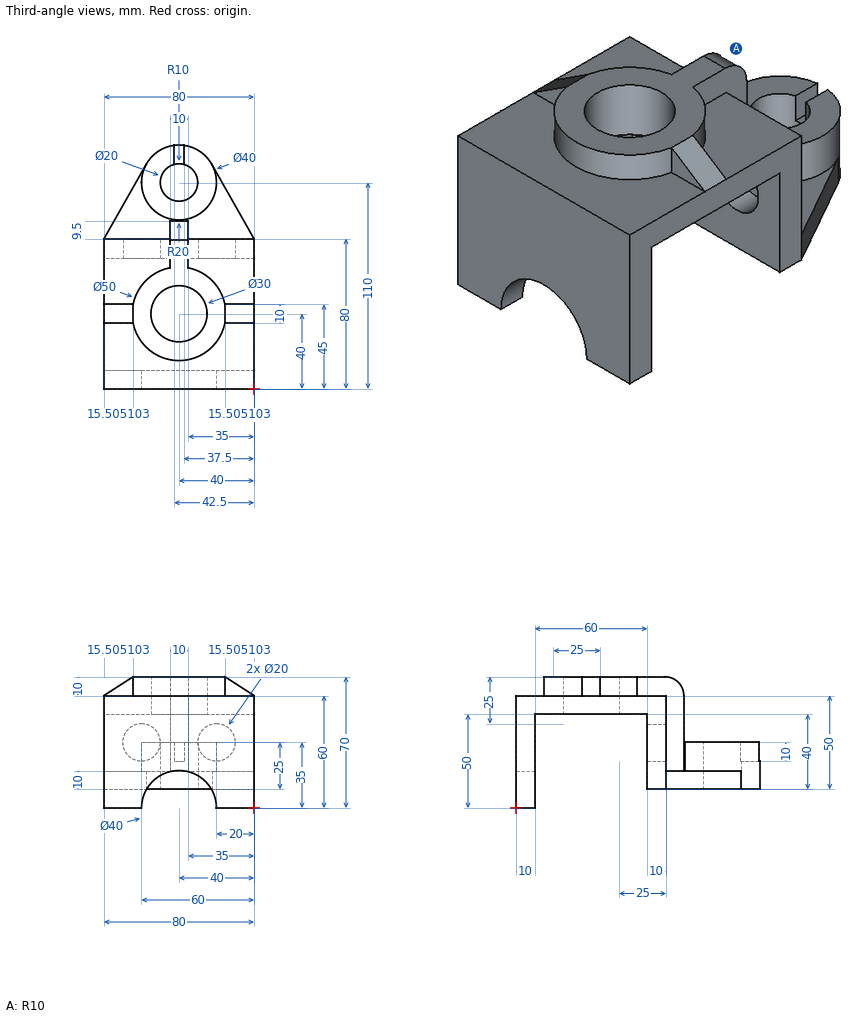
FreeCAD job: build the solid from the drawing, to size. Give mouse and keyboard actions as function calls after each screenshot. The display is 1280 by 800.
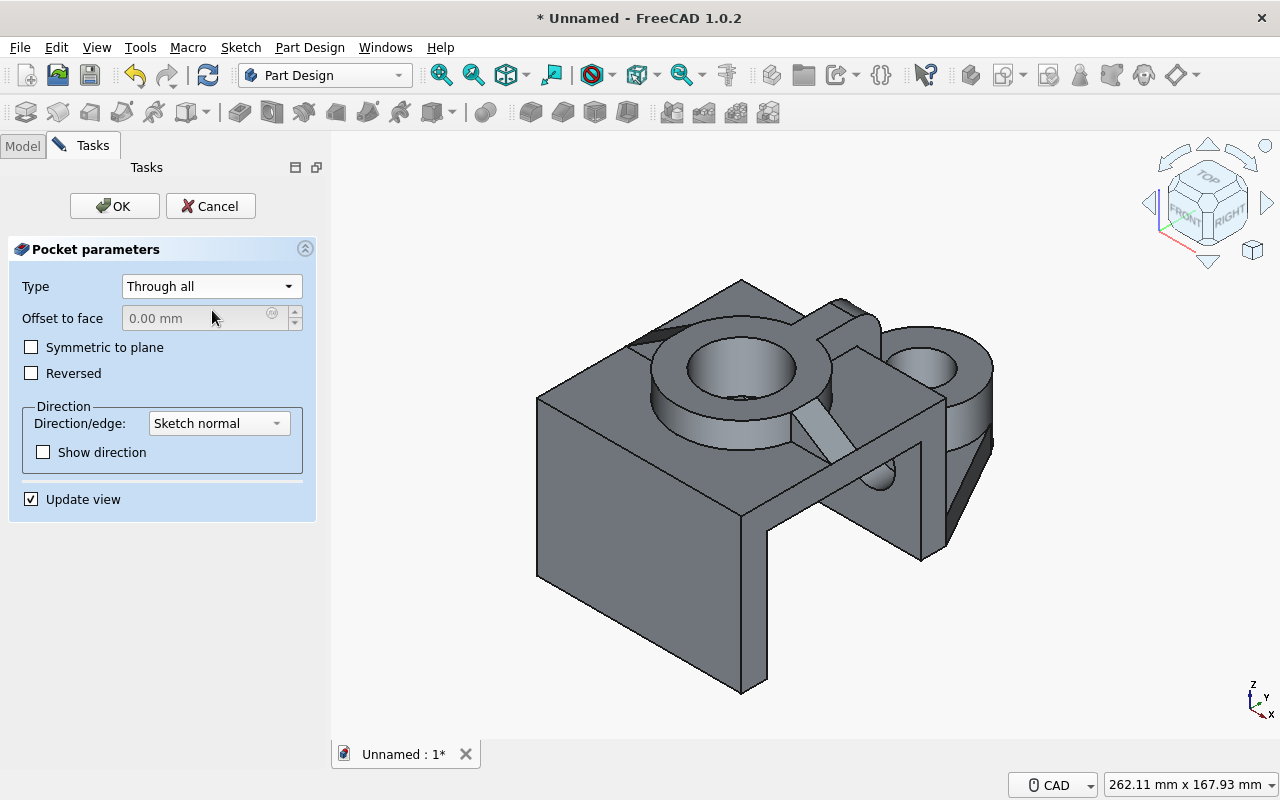
click(115, 206)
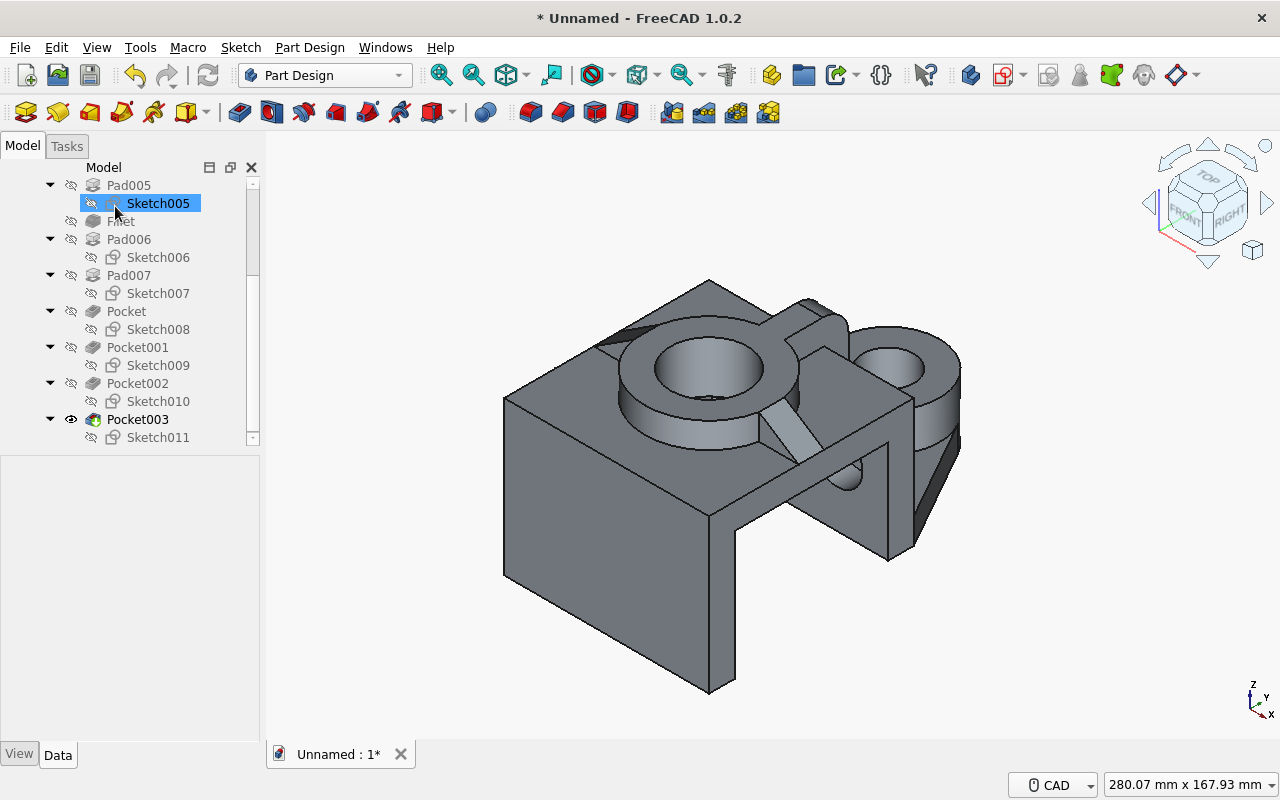
click(888, 334)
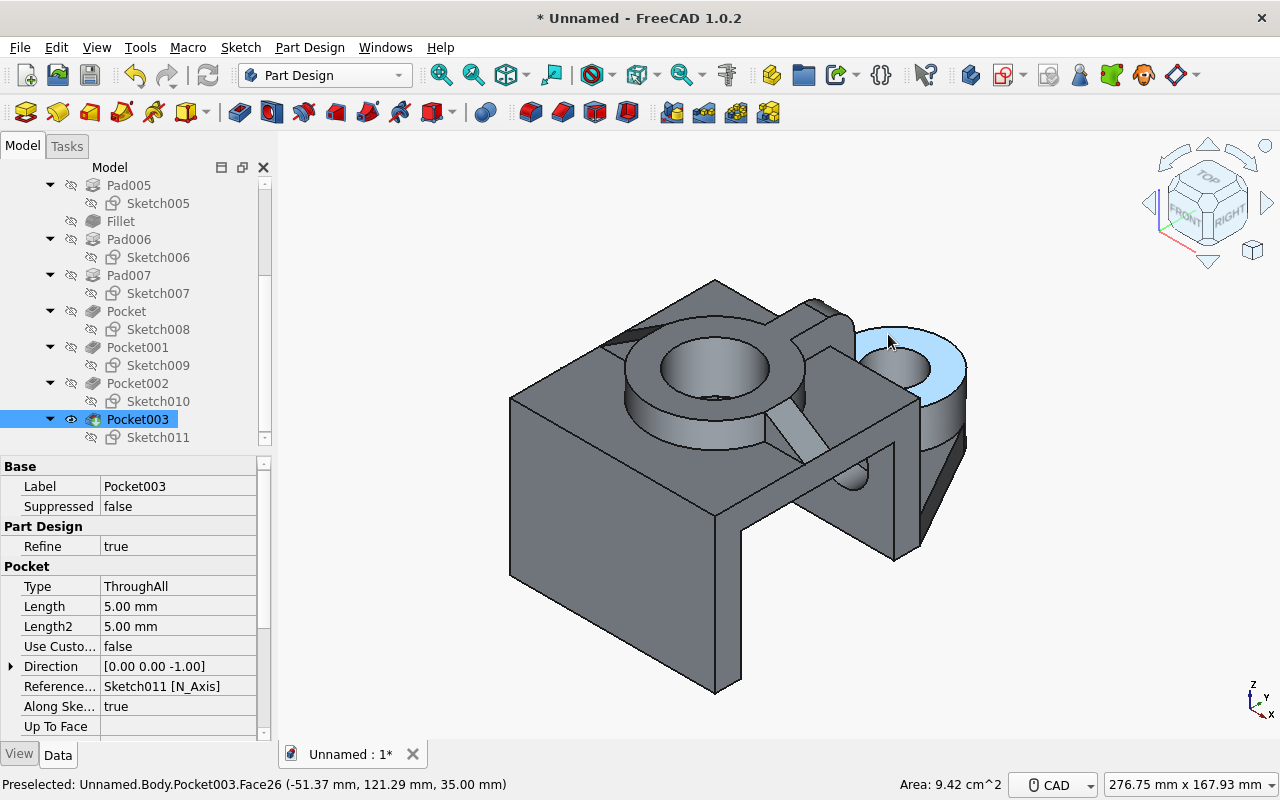
click(1004, 76)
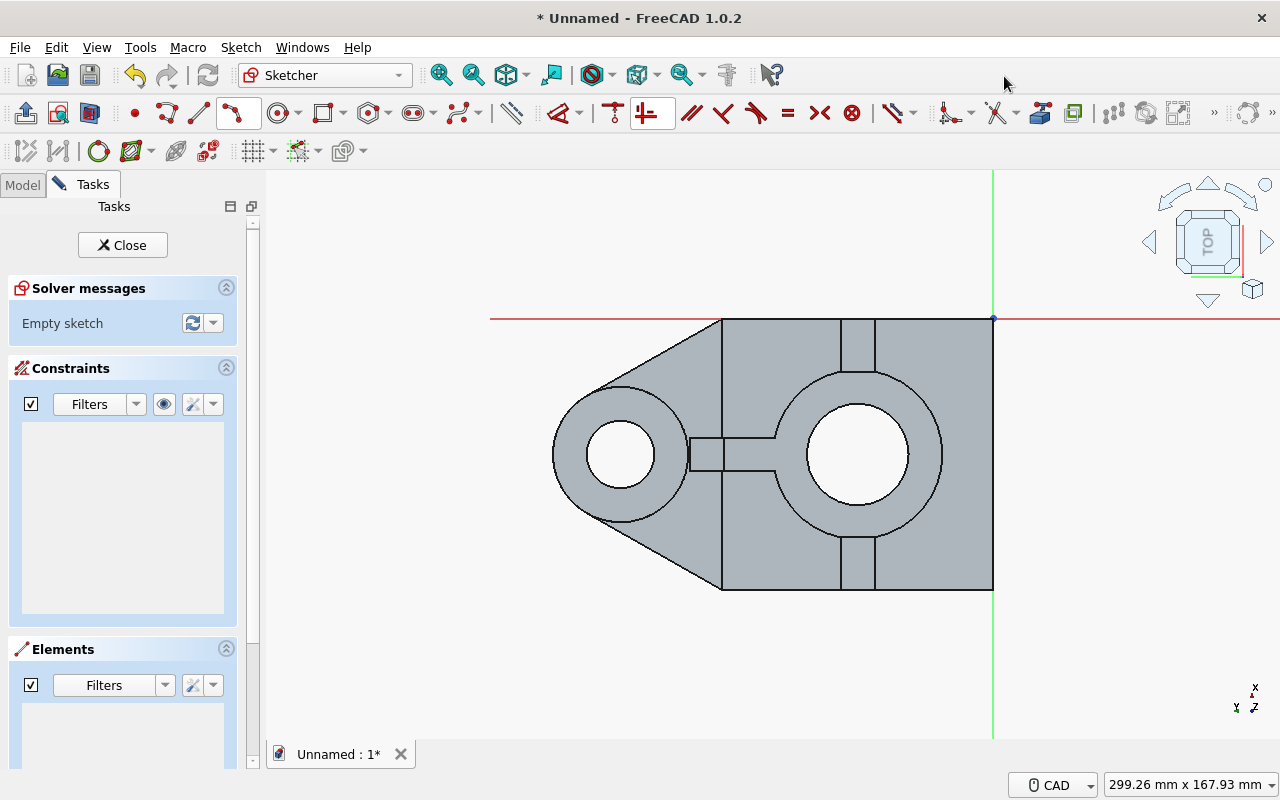
click(90, 114)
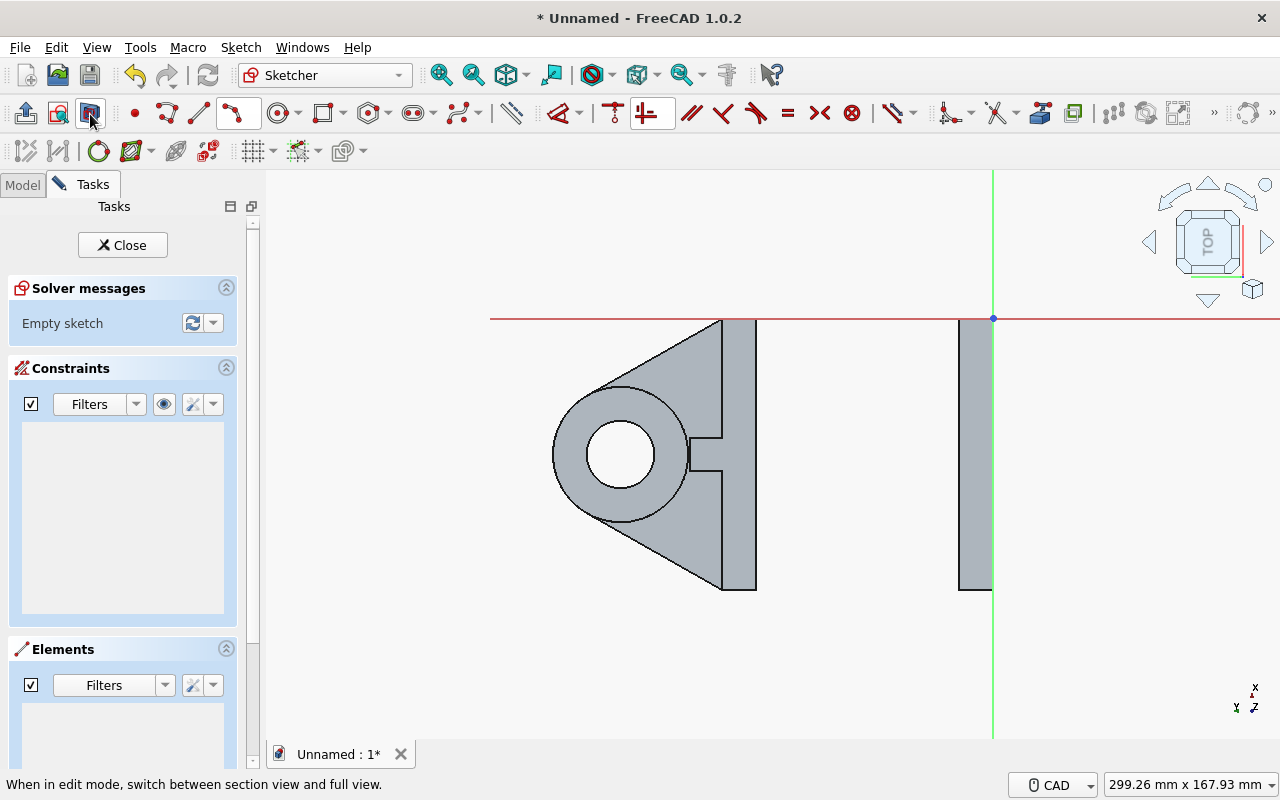
scroll(562, 455, up, 14)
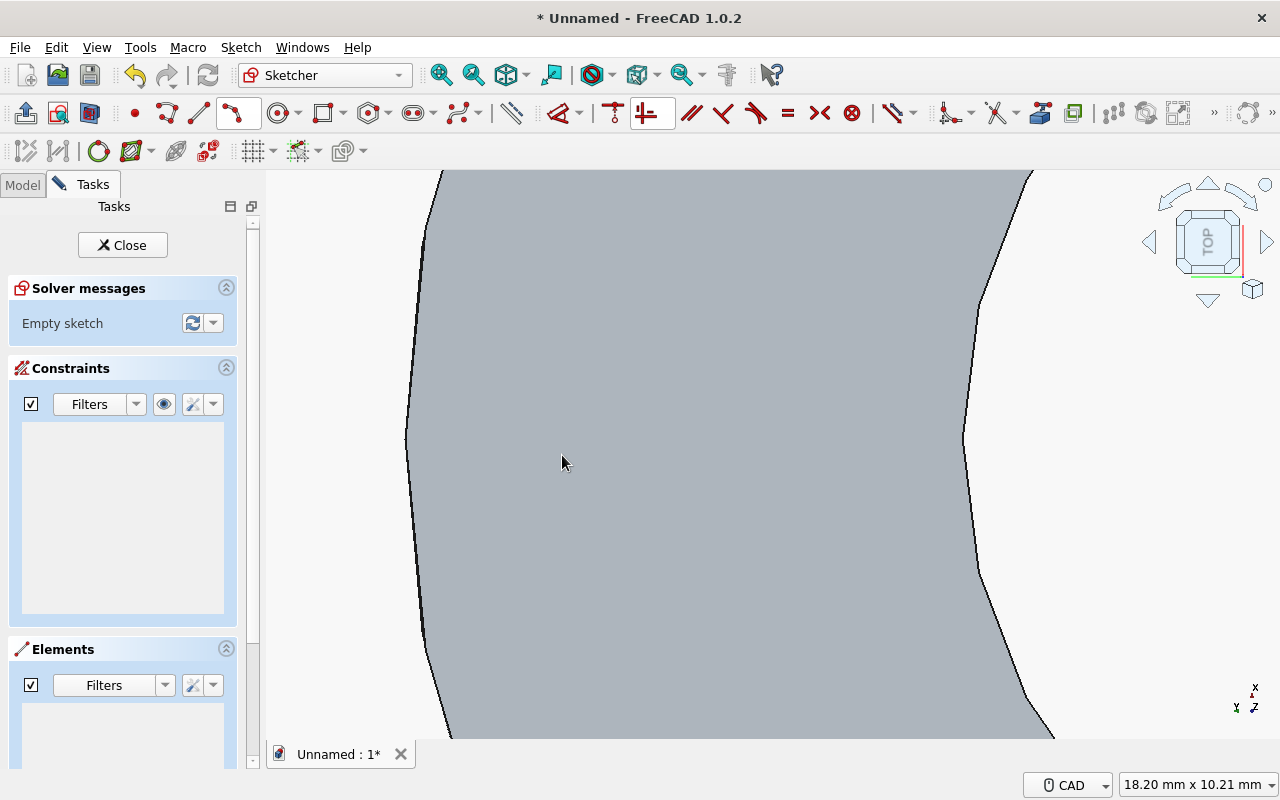
click(200, 114)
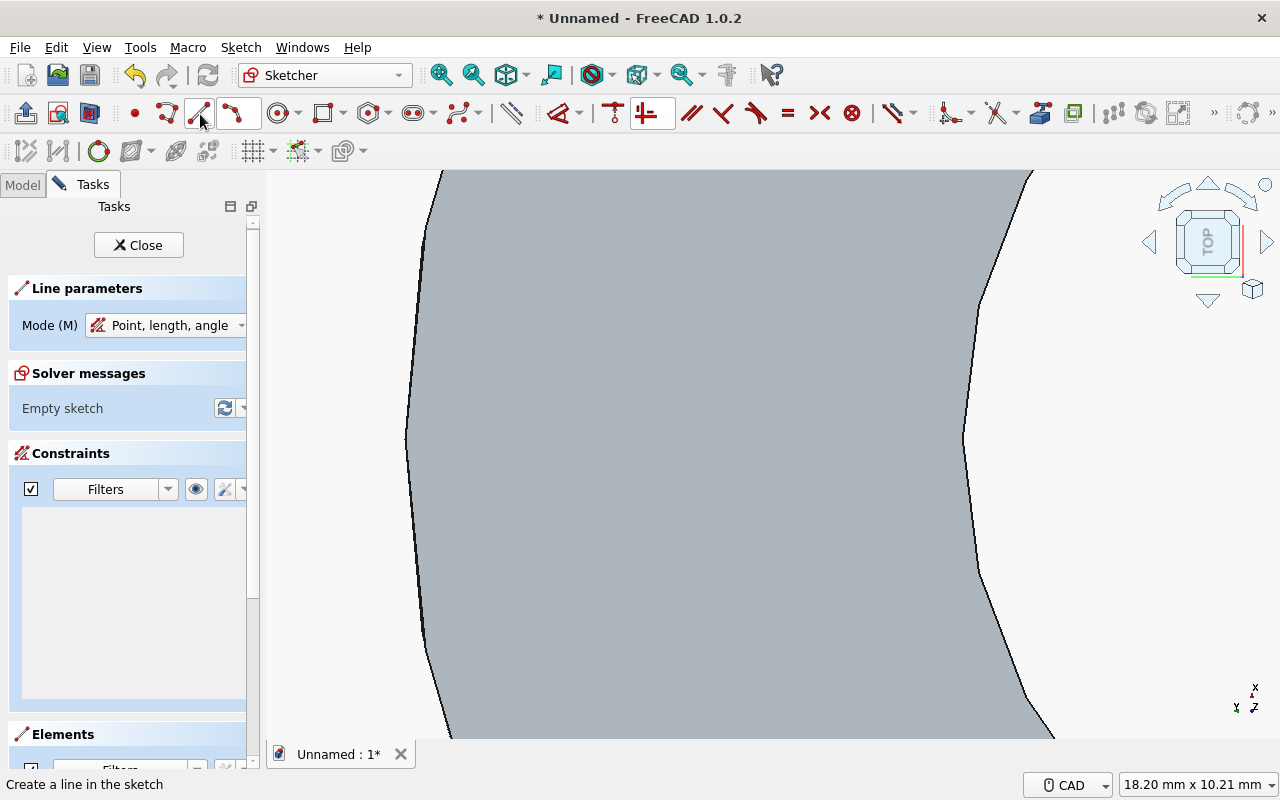
click(414, 578)
click(980, 578)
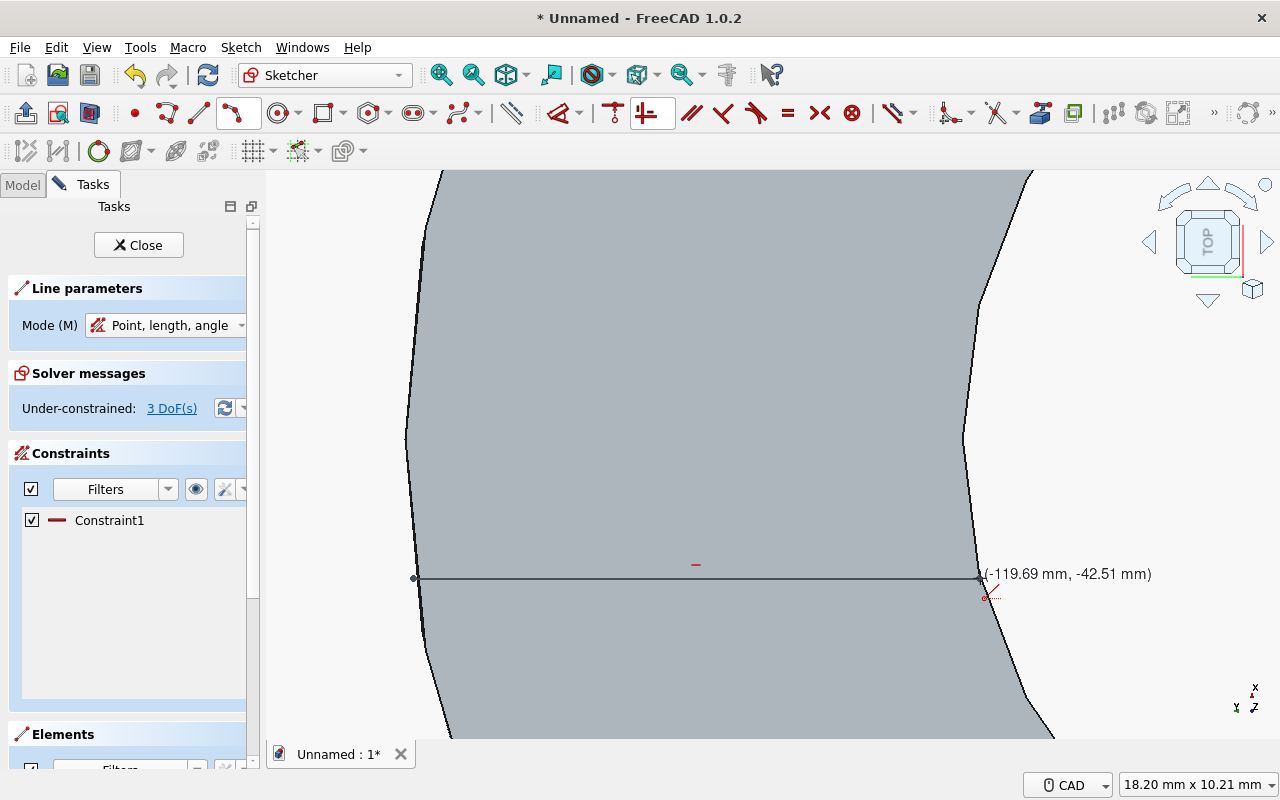
click(980, 300)
click(414, 300)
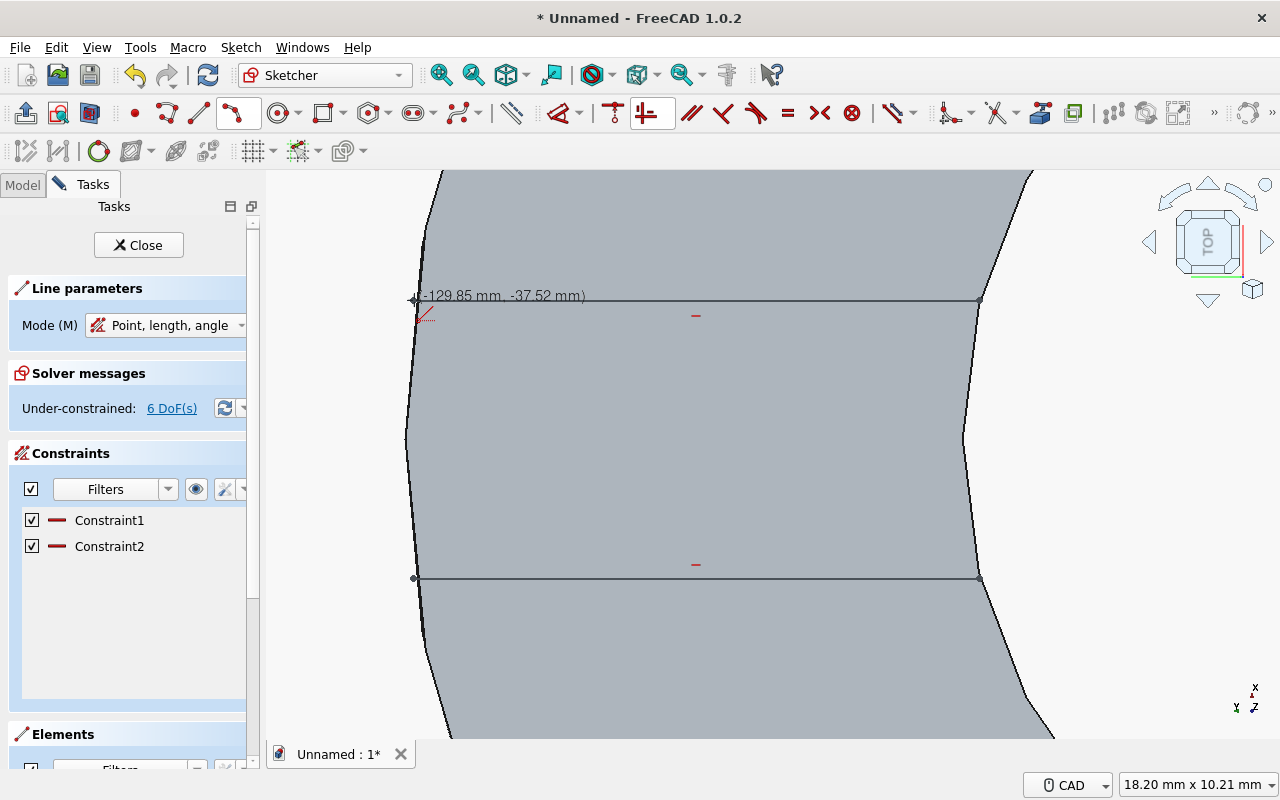
click(232, 114)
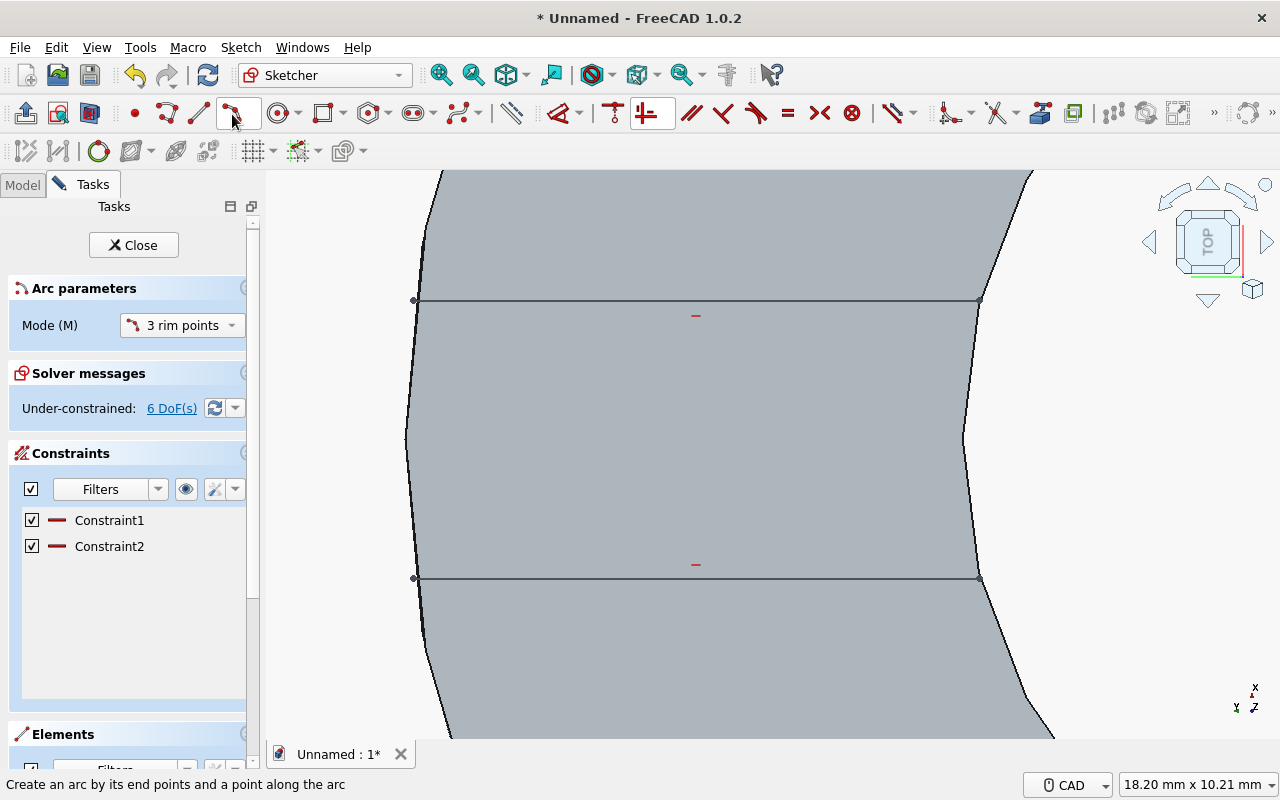
click(980, 579)
click(980, 301)
click(963, 439)